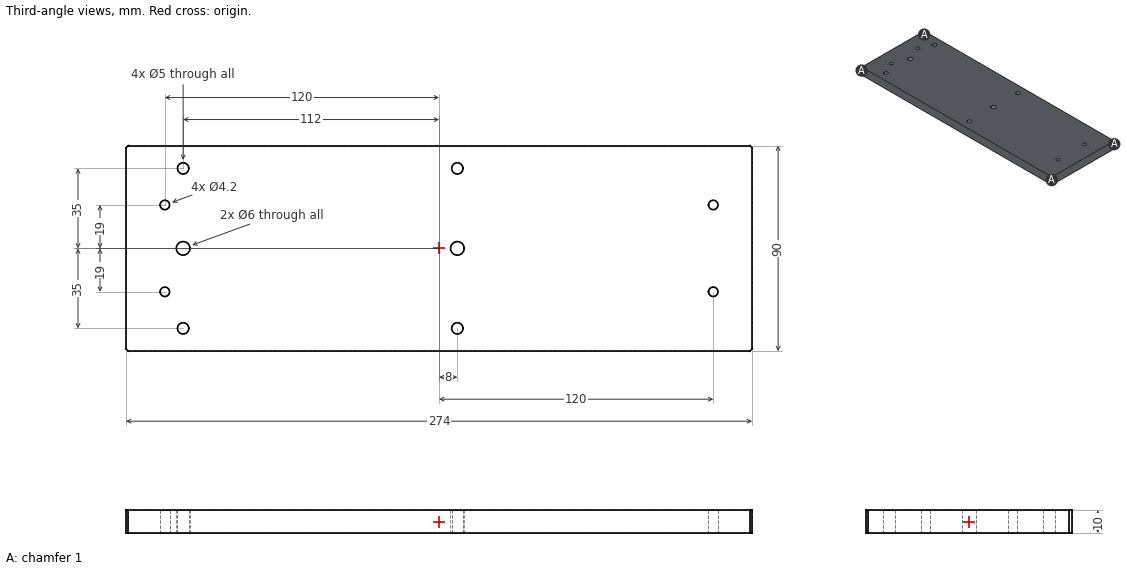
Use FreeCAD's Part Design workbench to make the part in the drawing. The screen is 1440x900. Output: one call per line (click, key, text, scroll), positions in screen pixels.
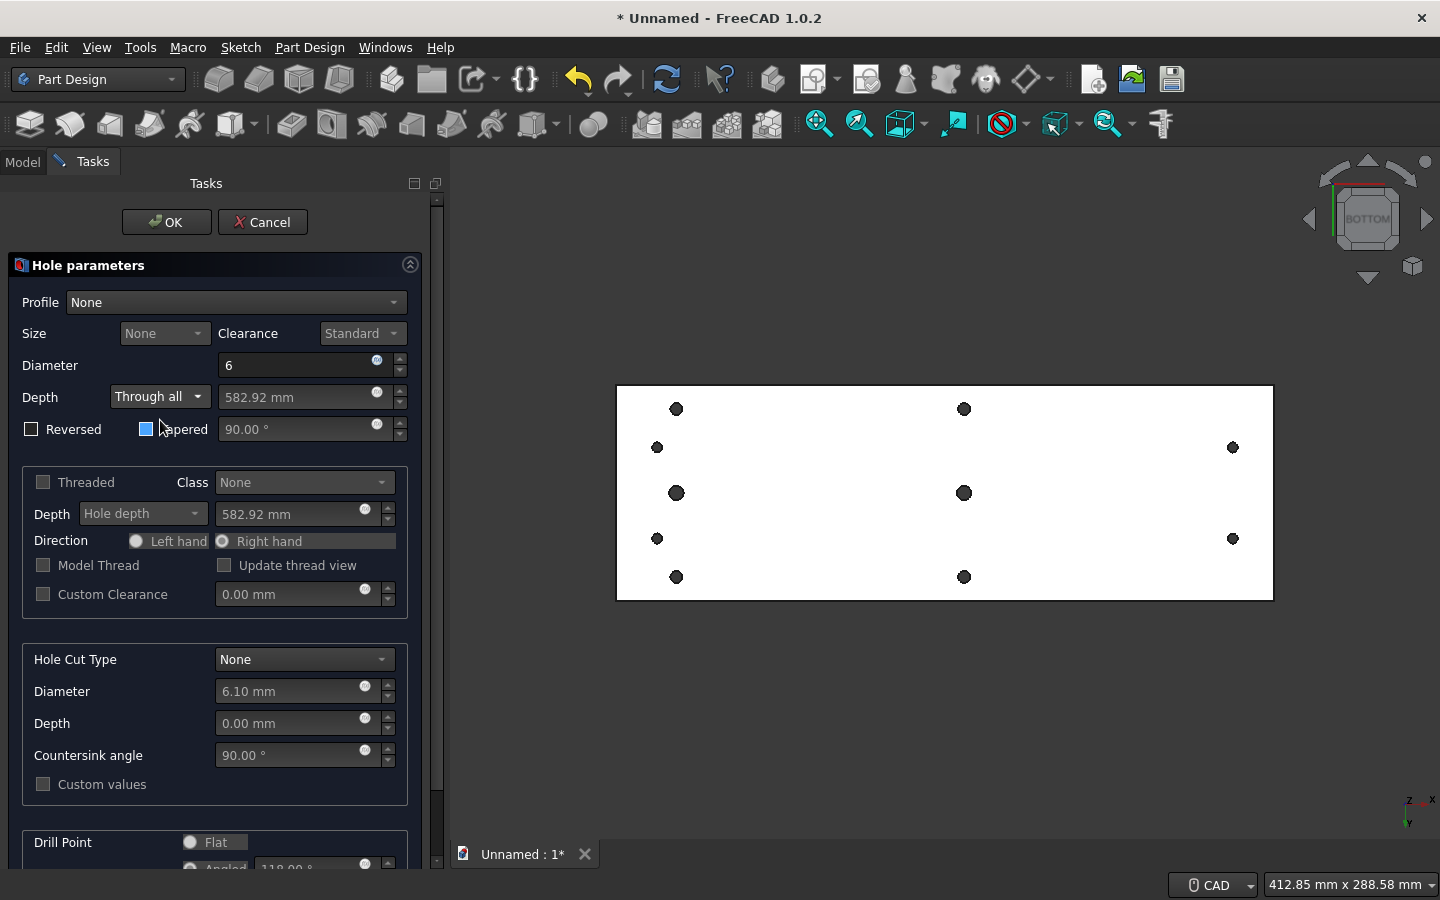
click(167, 222)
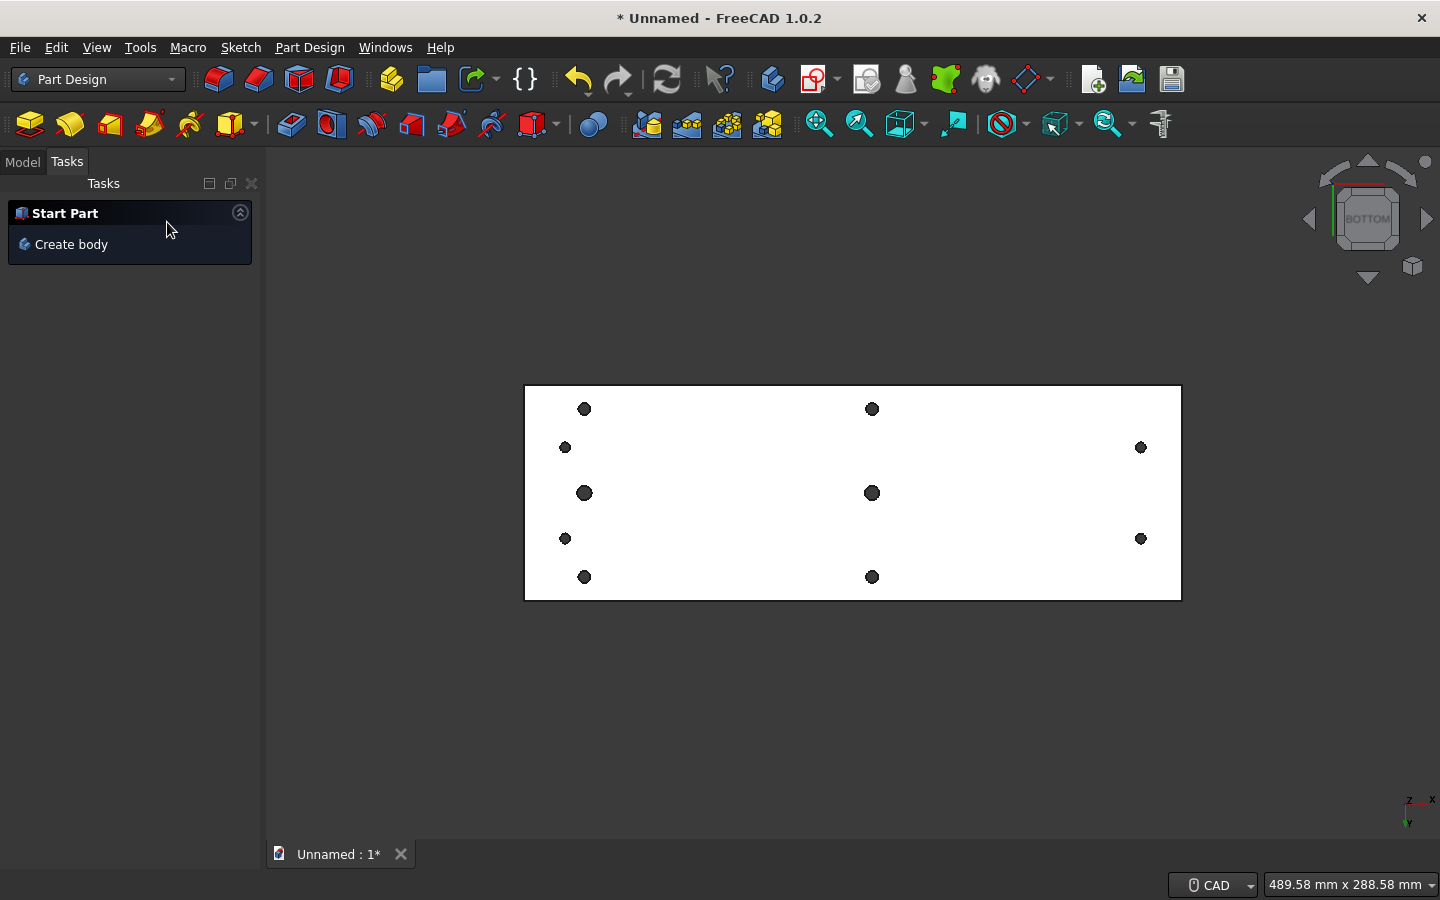
key(0)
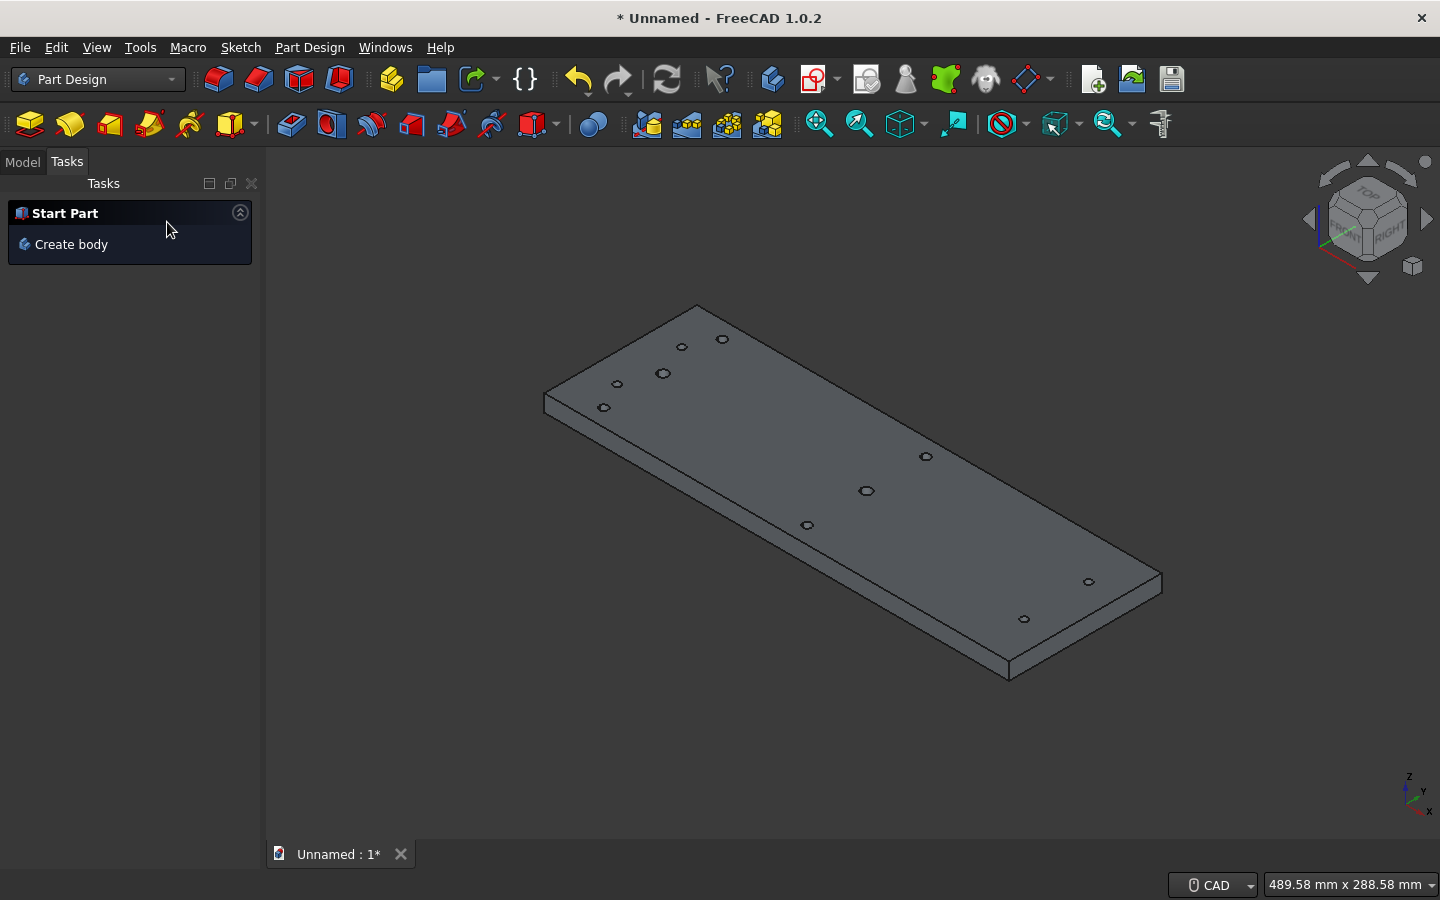
click(1009, 670)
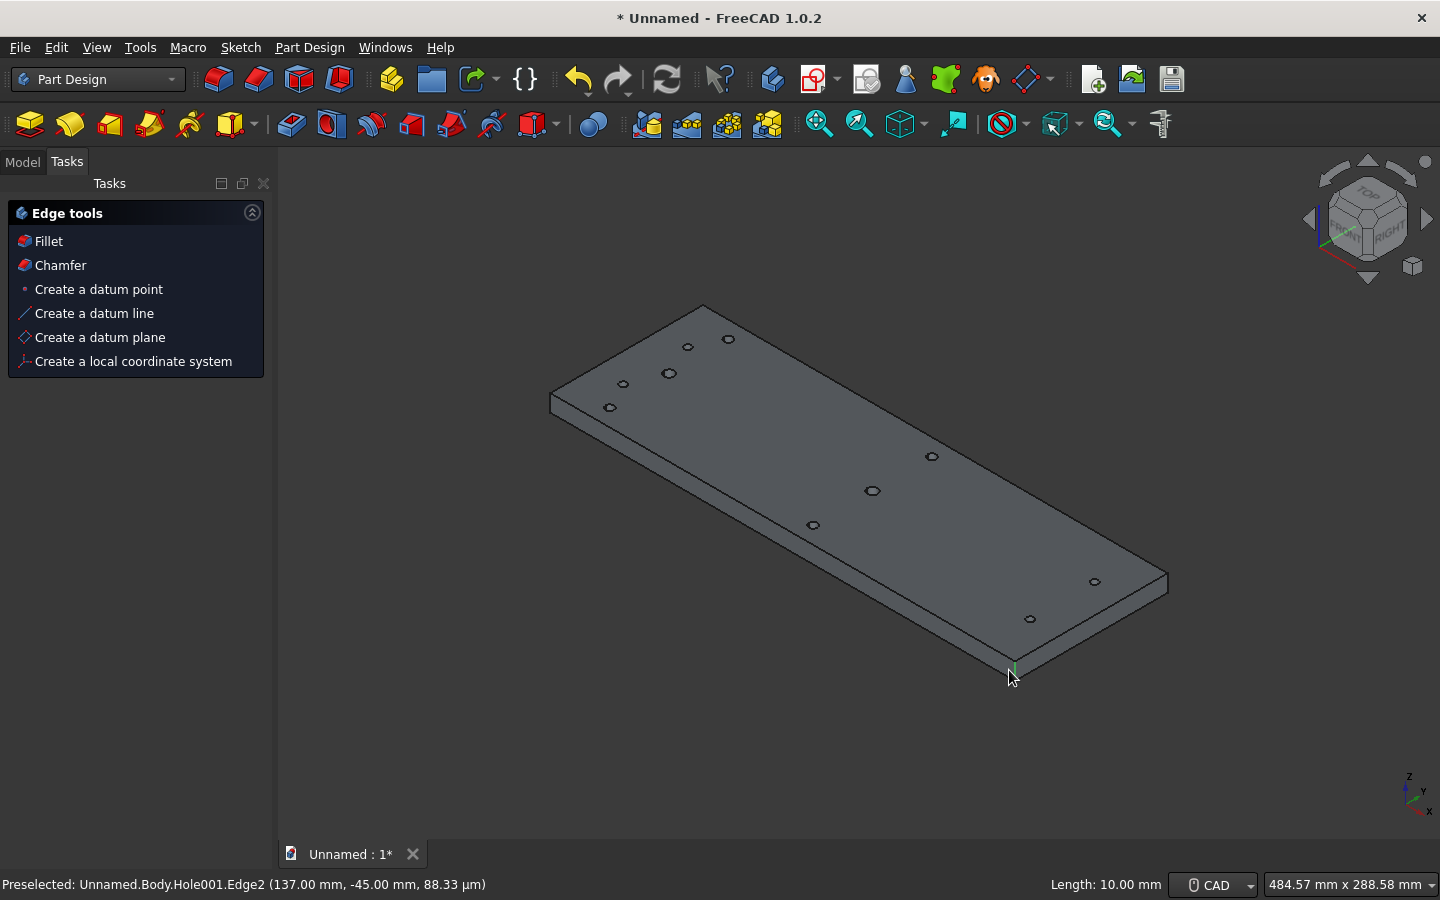
key(2)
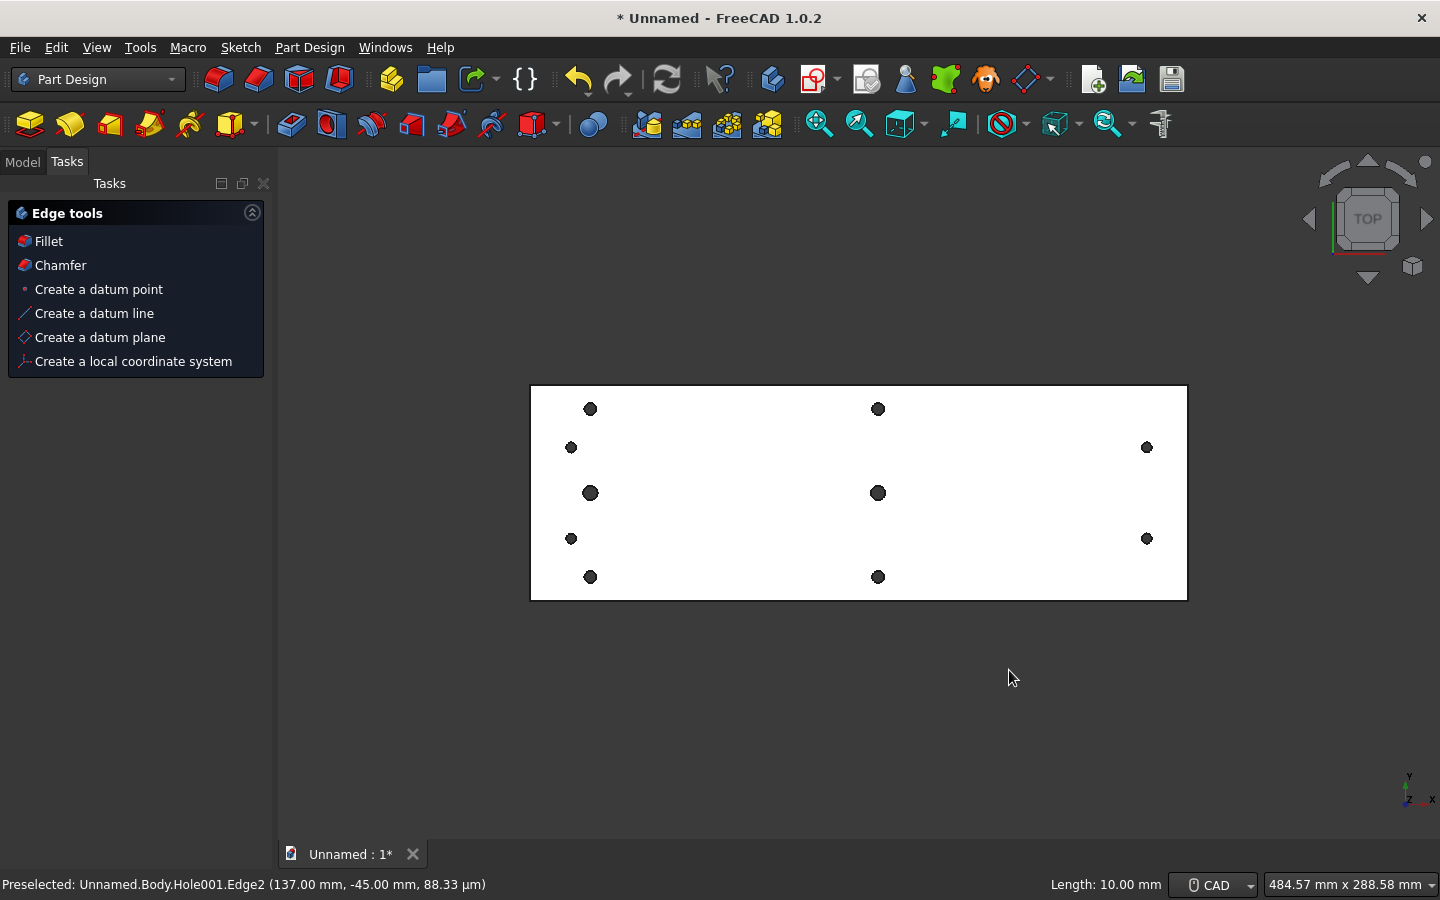
key(1)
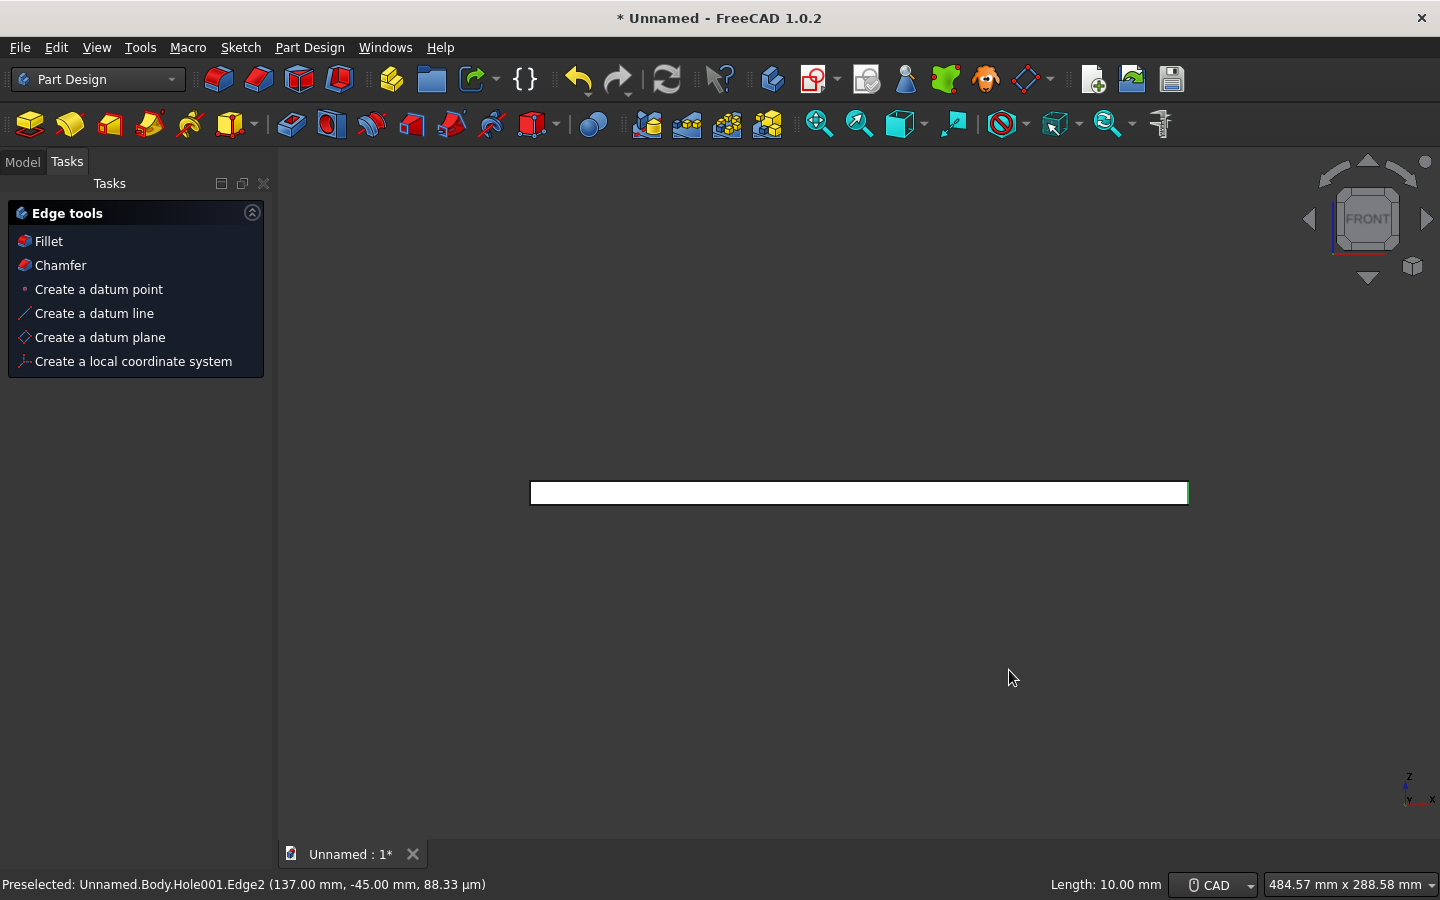
click(530, 492, ctrl)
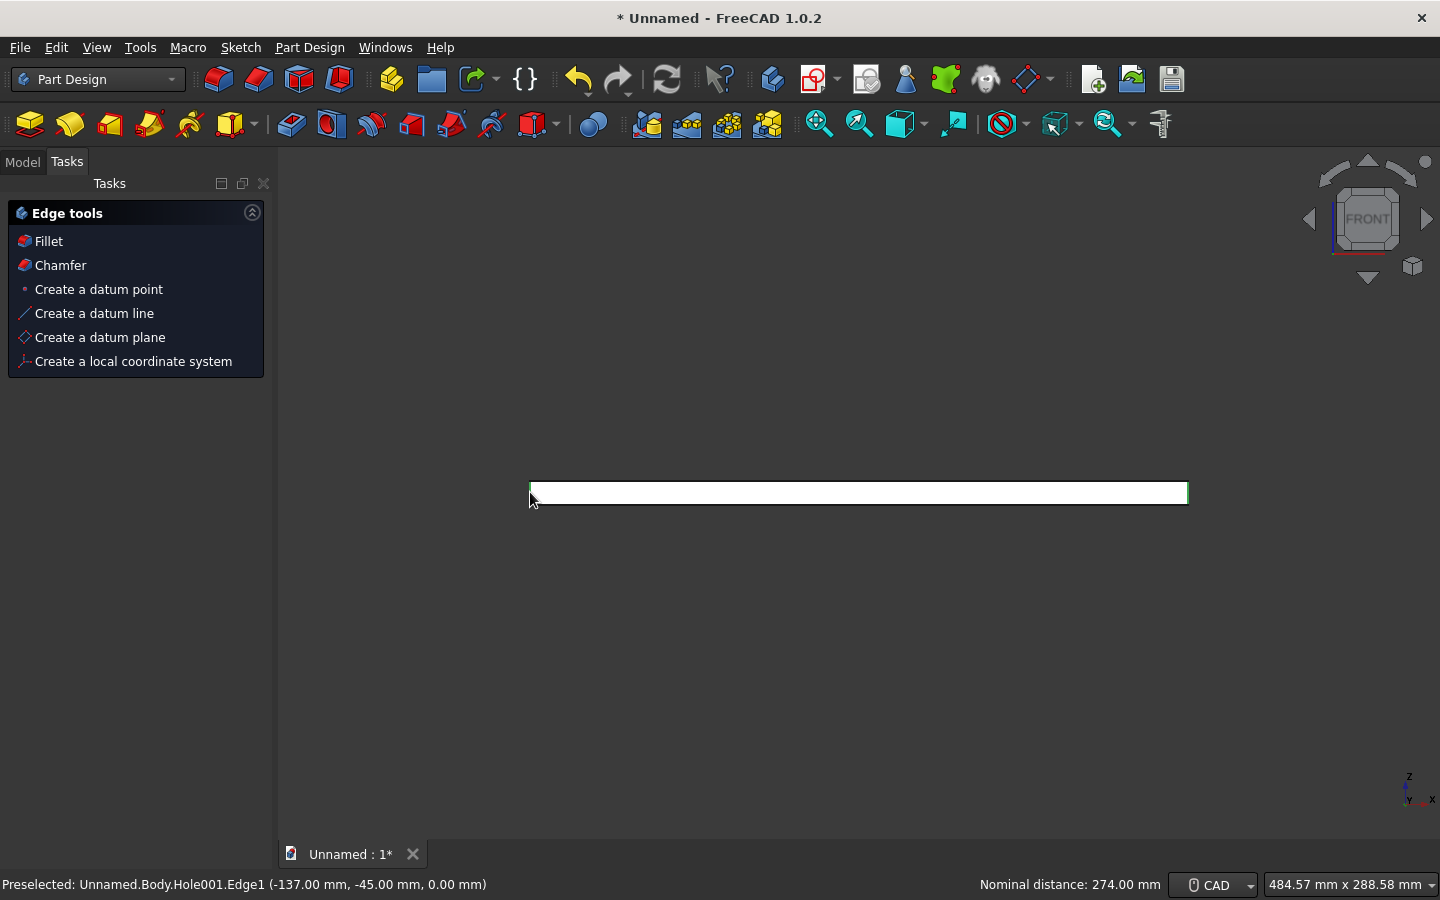
key(3)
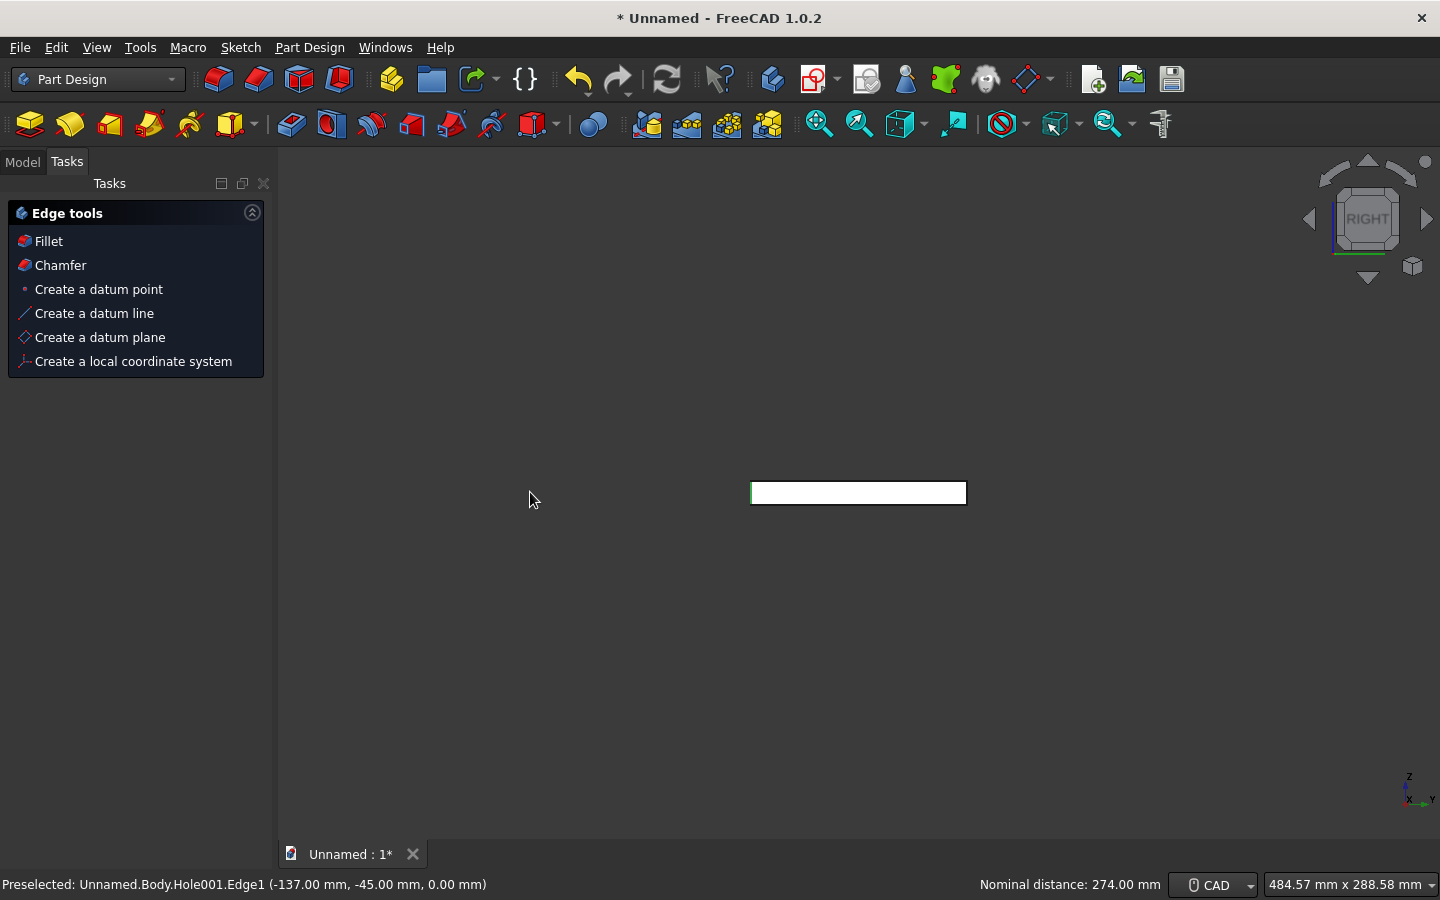
key(v)
key(f)